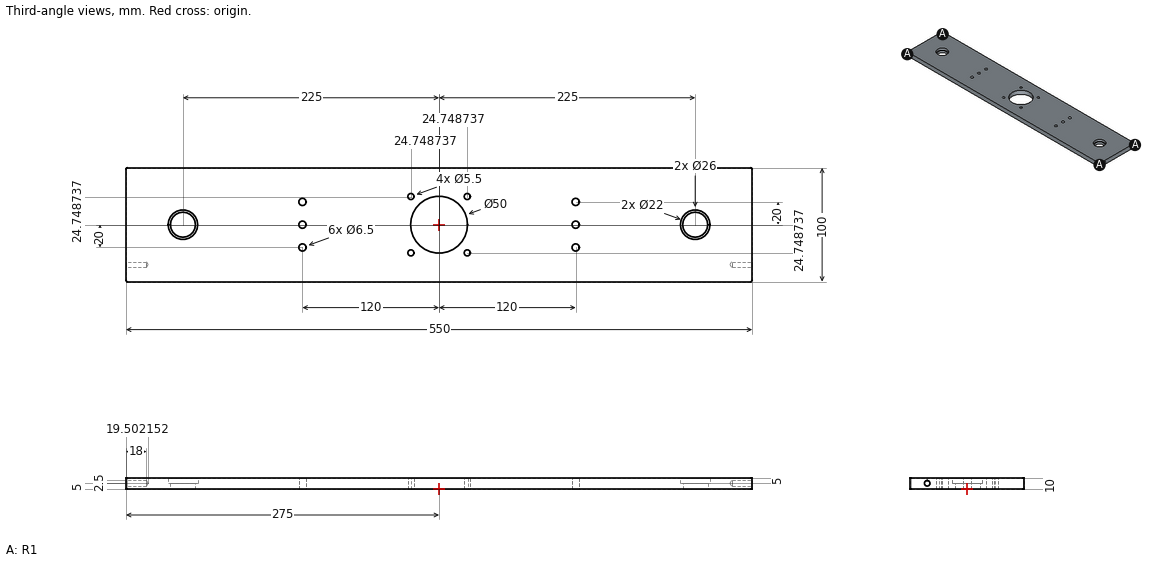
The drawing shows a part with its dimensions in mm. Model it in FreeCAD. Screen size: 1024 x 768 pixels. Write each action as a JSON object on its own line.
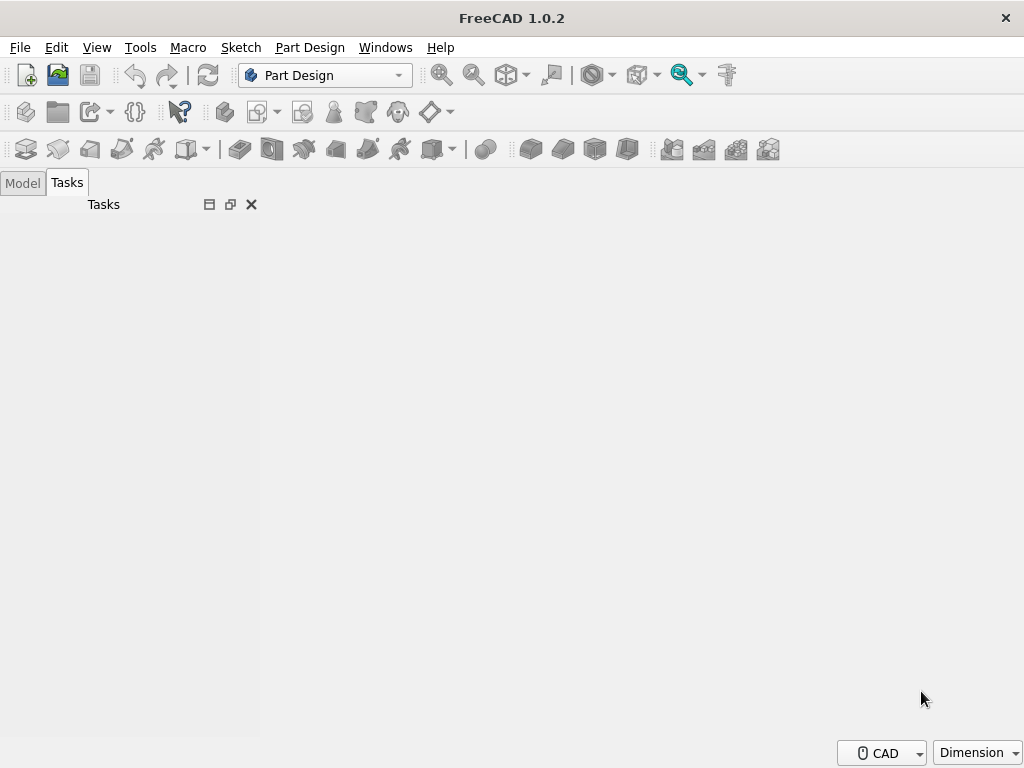
{"action": "left_click", "coordinate": [26, 76]}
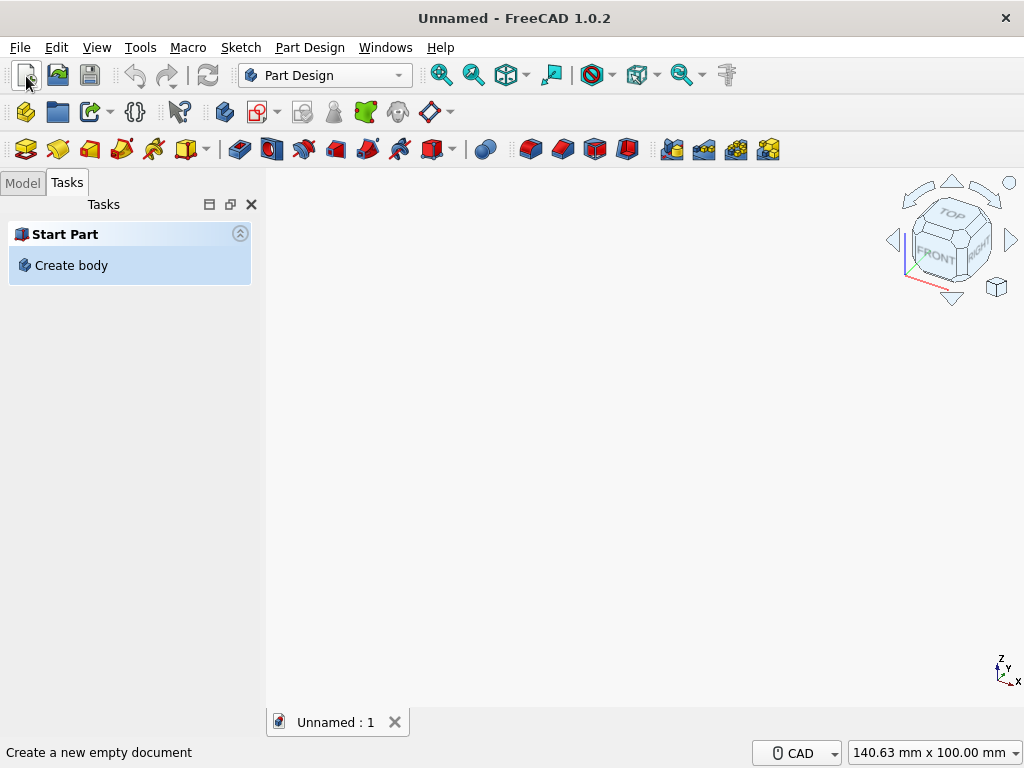
{"action": "left_click", "coordinate": [258, 112]}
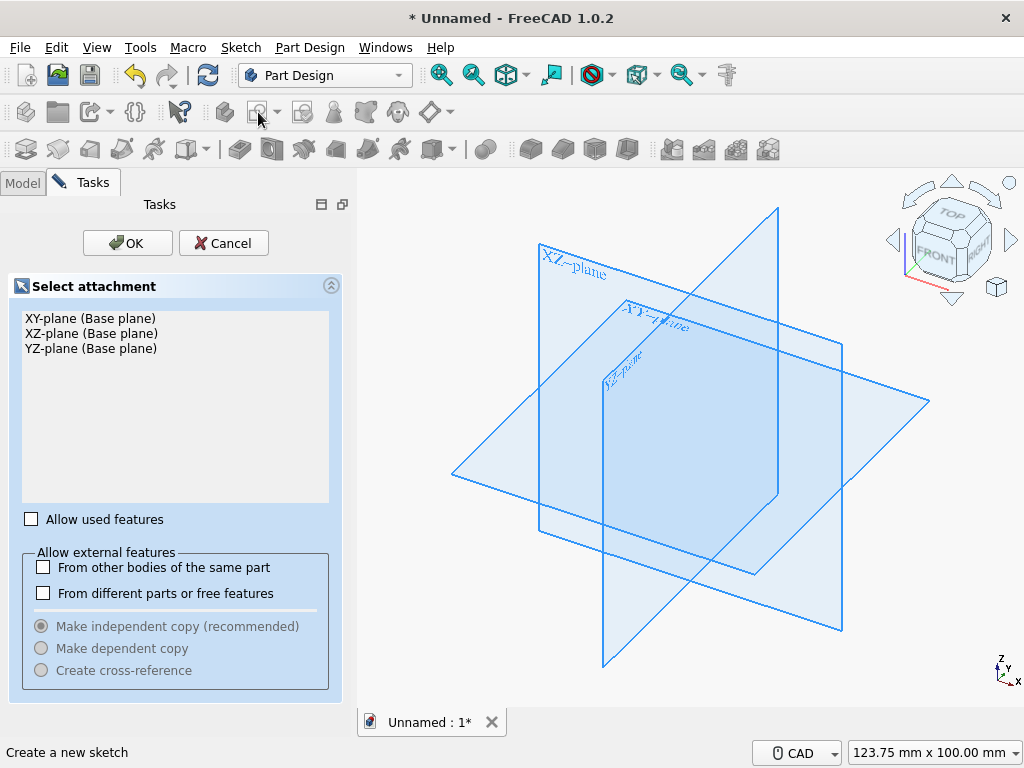
{"action": "left_click", "coordinate": [82, 318]}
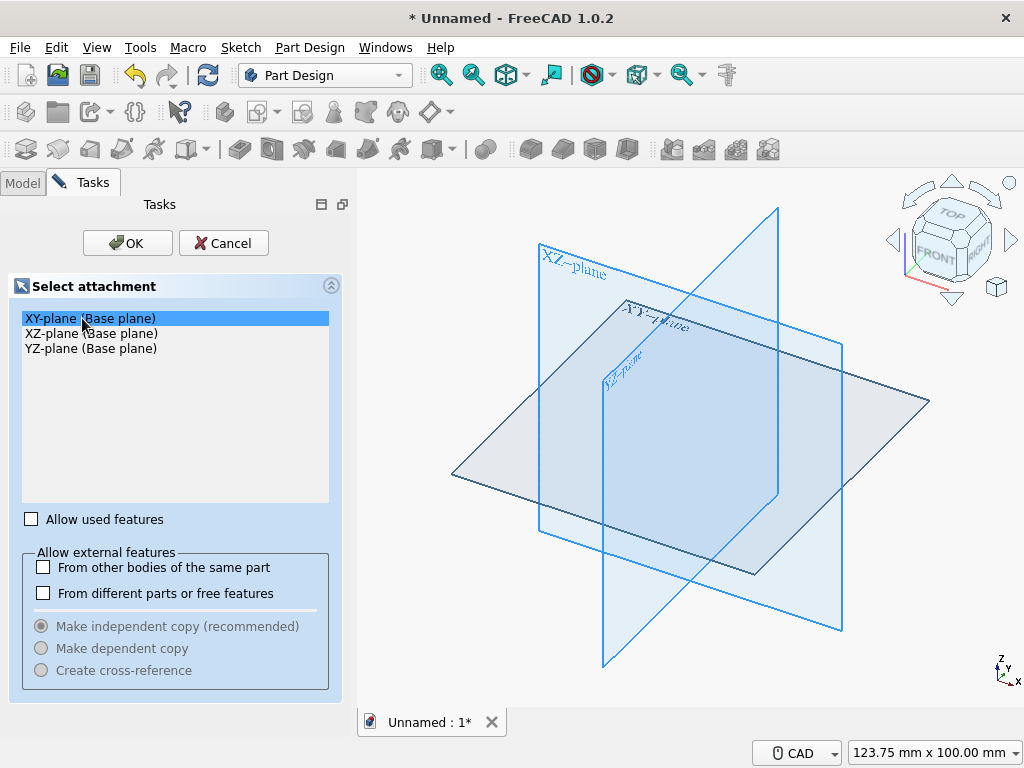
{"action": "left_click", "coordinate": [128, 243]}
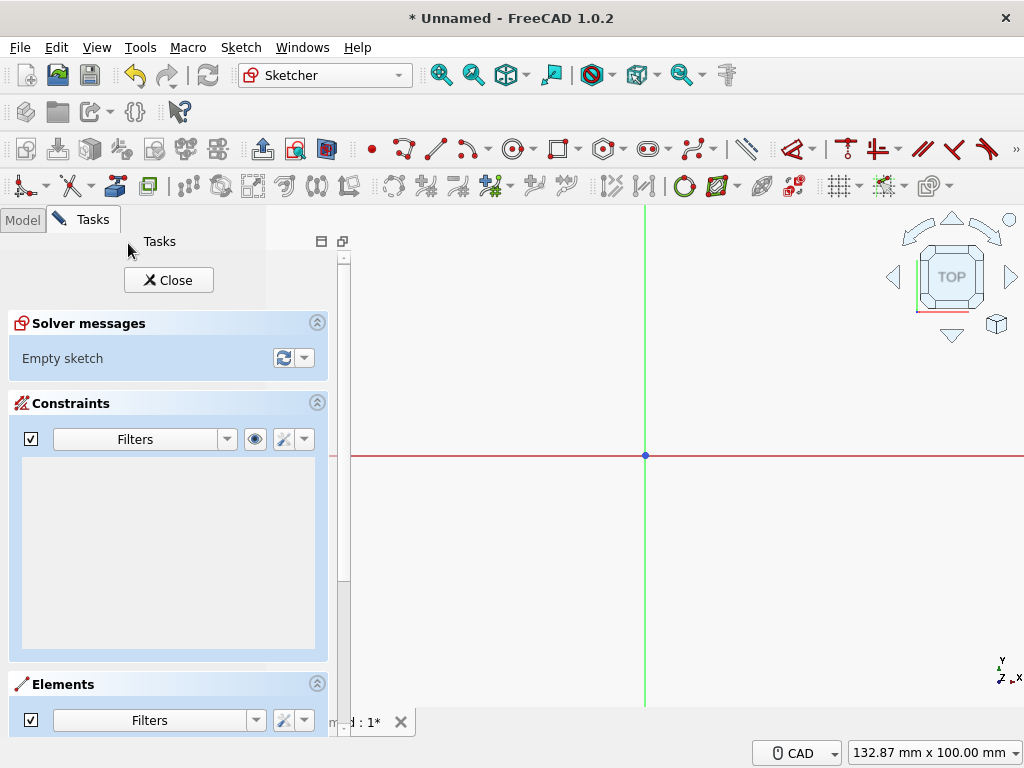
{"action": "scroll", "coordinate": [566, 456], "scroll_direction": "down", "scroll_amount": 10}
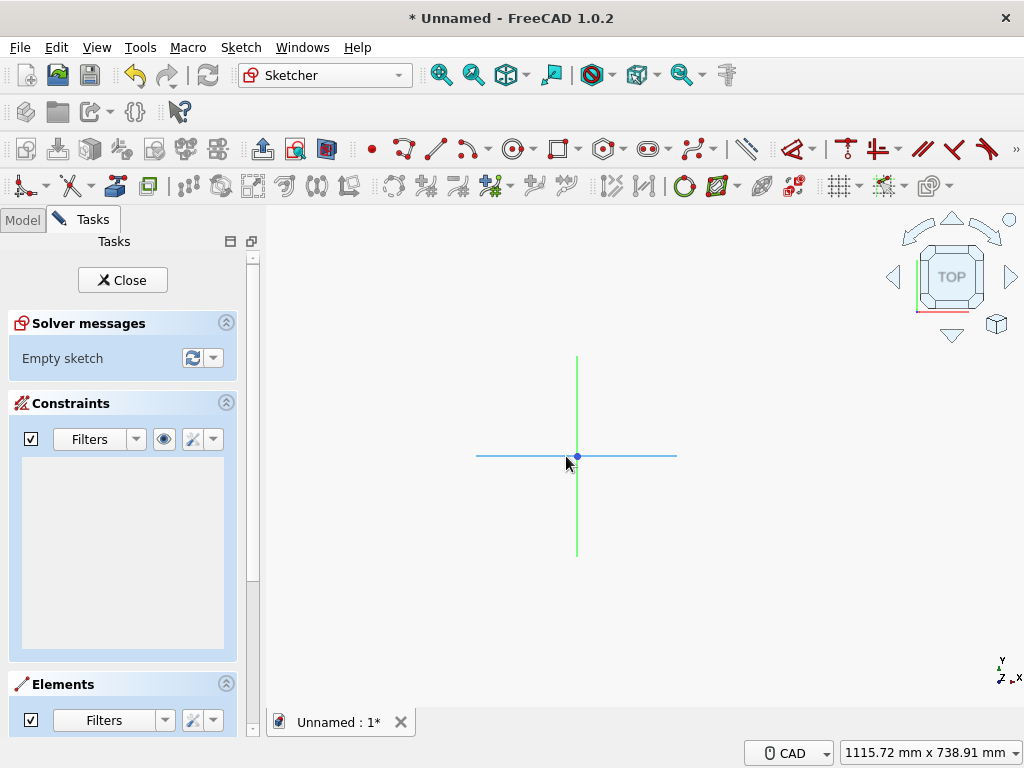
{"action": "key", "text": "g v"}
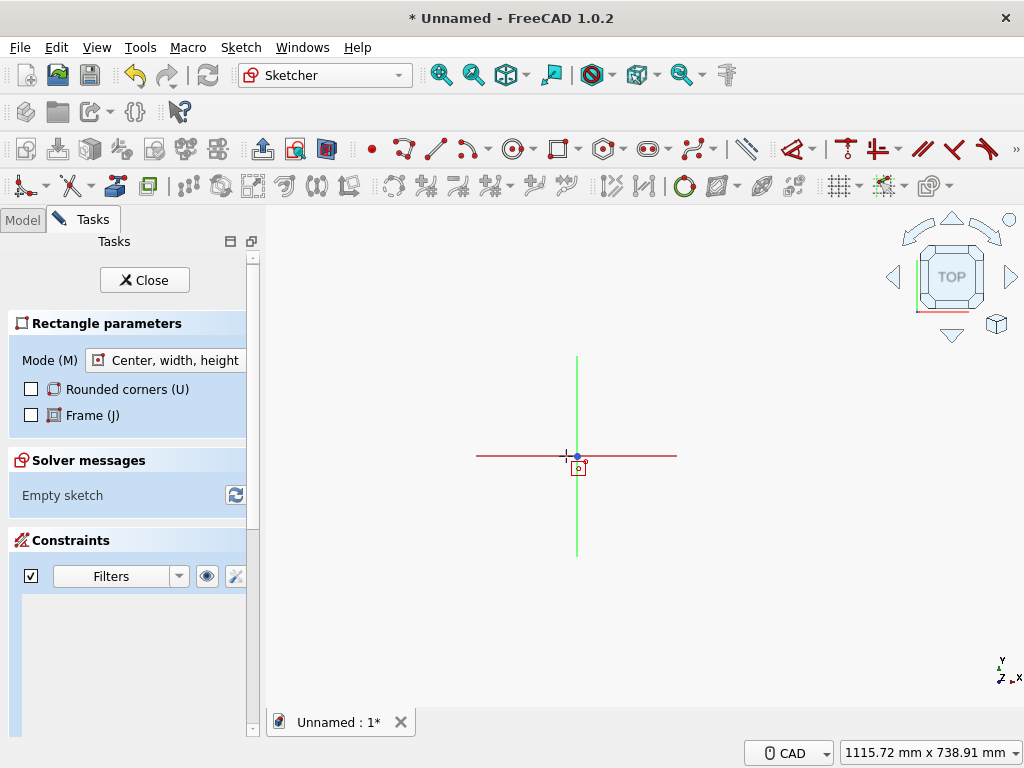
{"action": "left_click", "coordinate": [577, 456]}
{"action": "left_click", "coordinate": [764, 422]}
{"action": "key", "text": "Escape"}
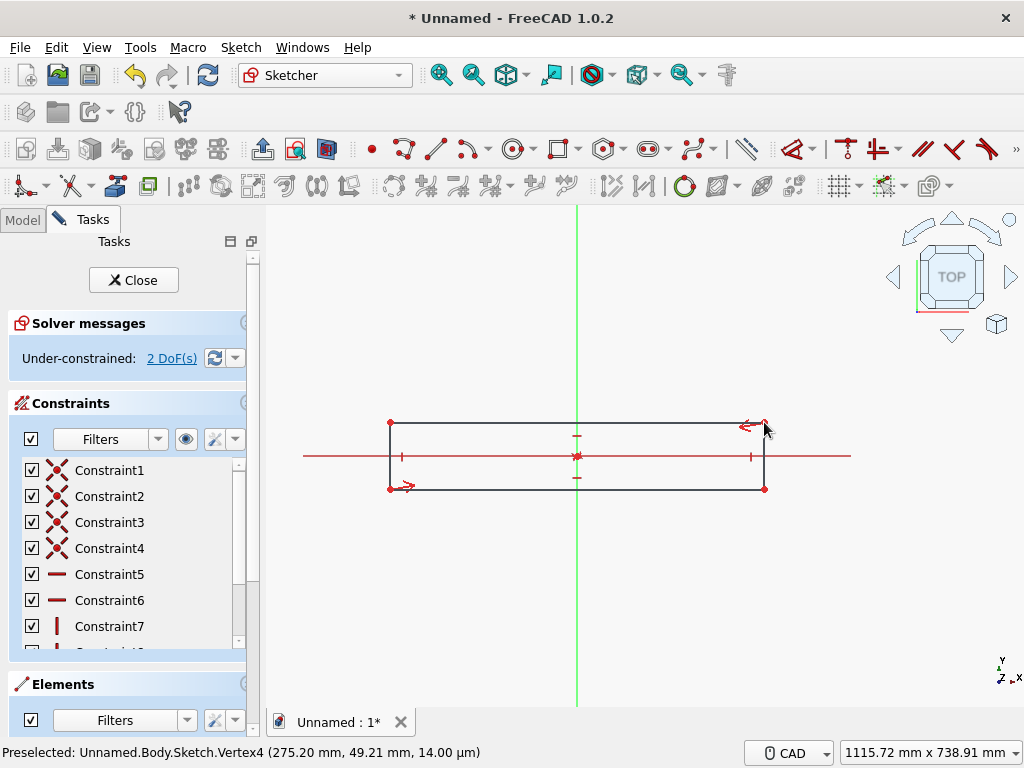
{"action": "key", "text": "d"}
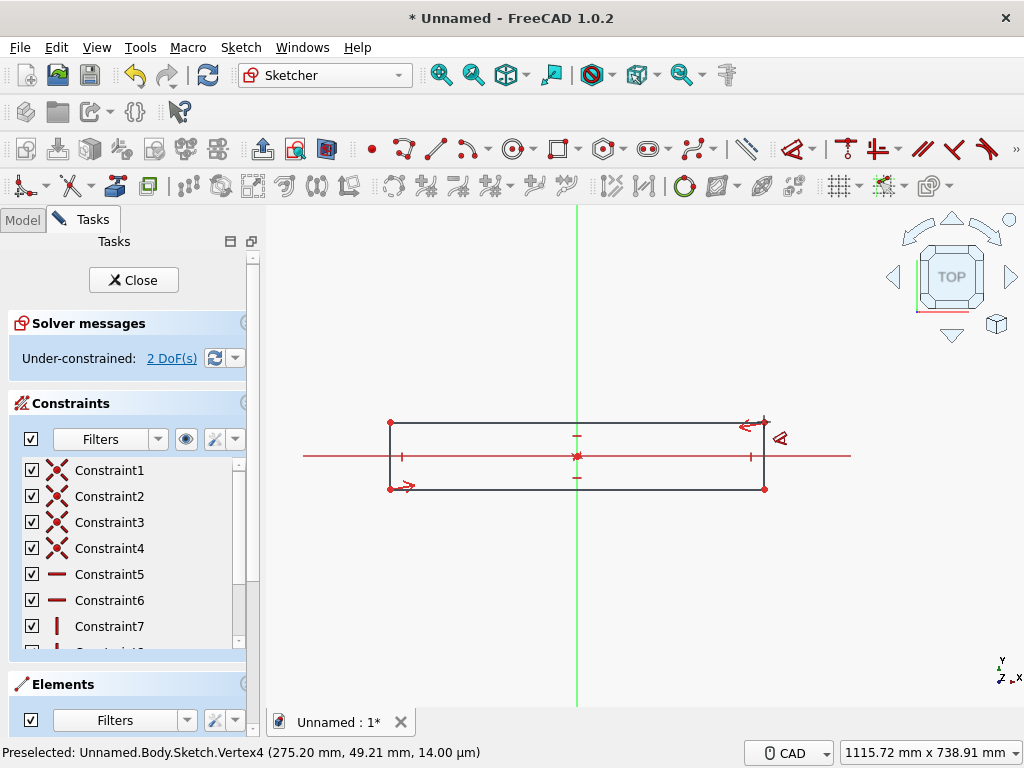
{"action": "left_click", "coordinate": [502, 490]}
{"action": "left_click", "coordinate": [491, 524]}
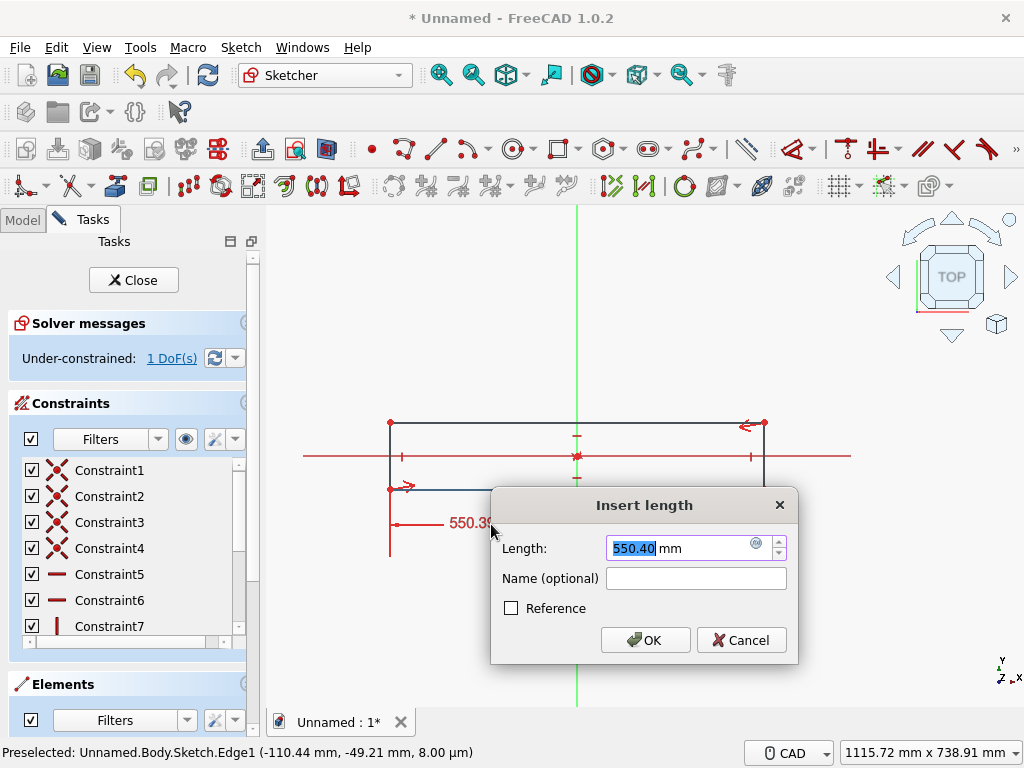
{"action": "type", "text": "550"}
{"action": "key", "text": "Return"}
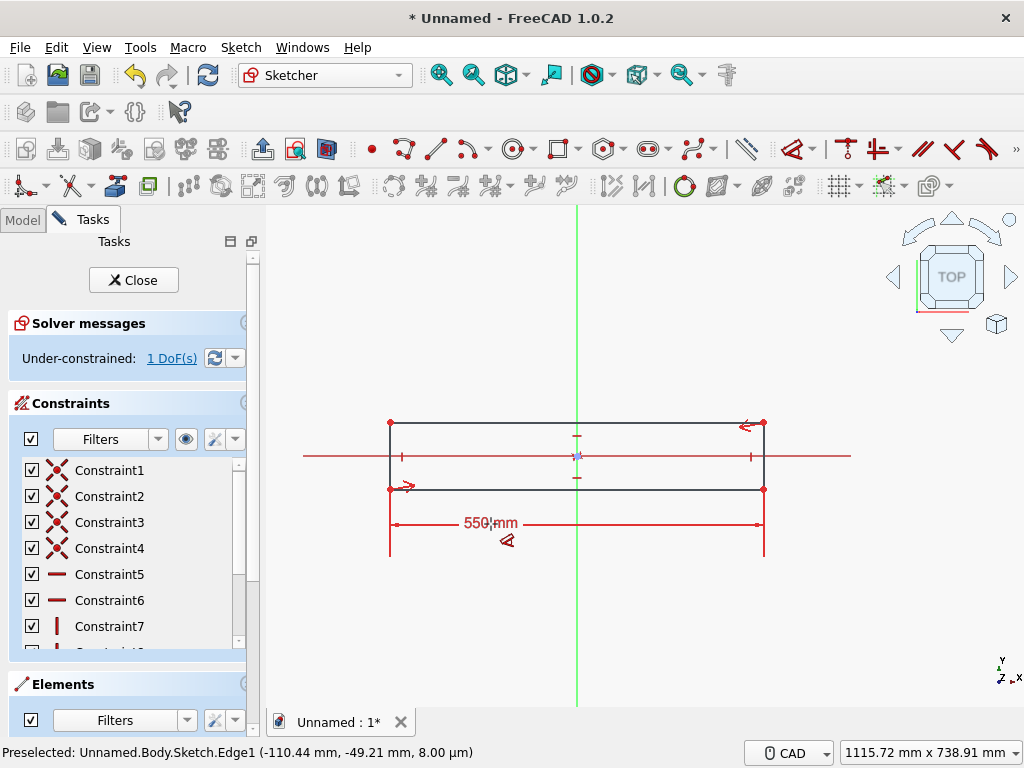
{"action": "left_click", "coordinate": [764, 470]}
{"action": "left_click", "coordinate": [798, 441]}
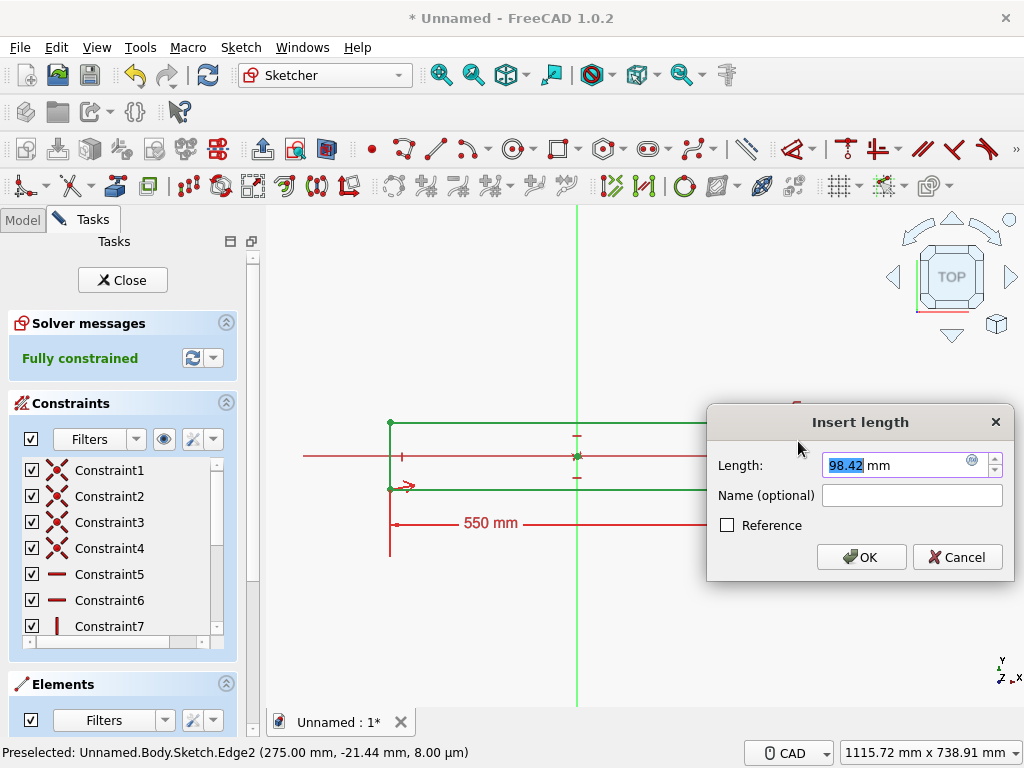
{"action": "type", "text": "100"}
{"action": "key", "text": "Return"}
{"action": "key", "text": "Escape"}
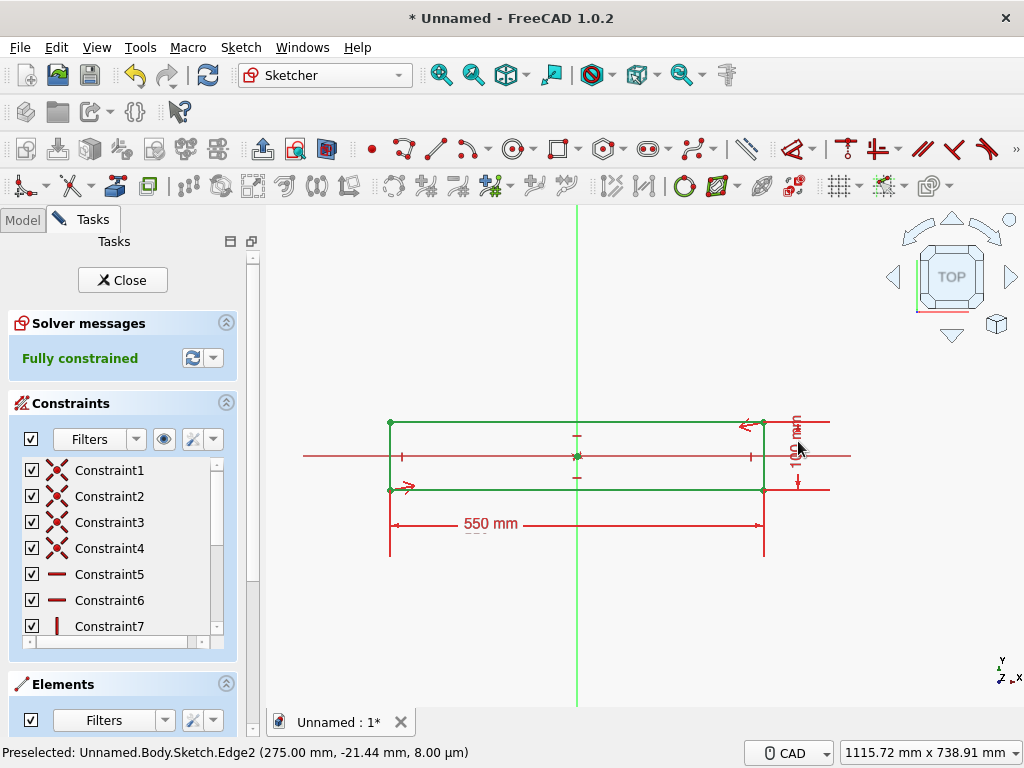
{"action": "left_click", "coordinate": [123, 280]}